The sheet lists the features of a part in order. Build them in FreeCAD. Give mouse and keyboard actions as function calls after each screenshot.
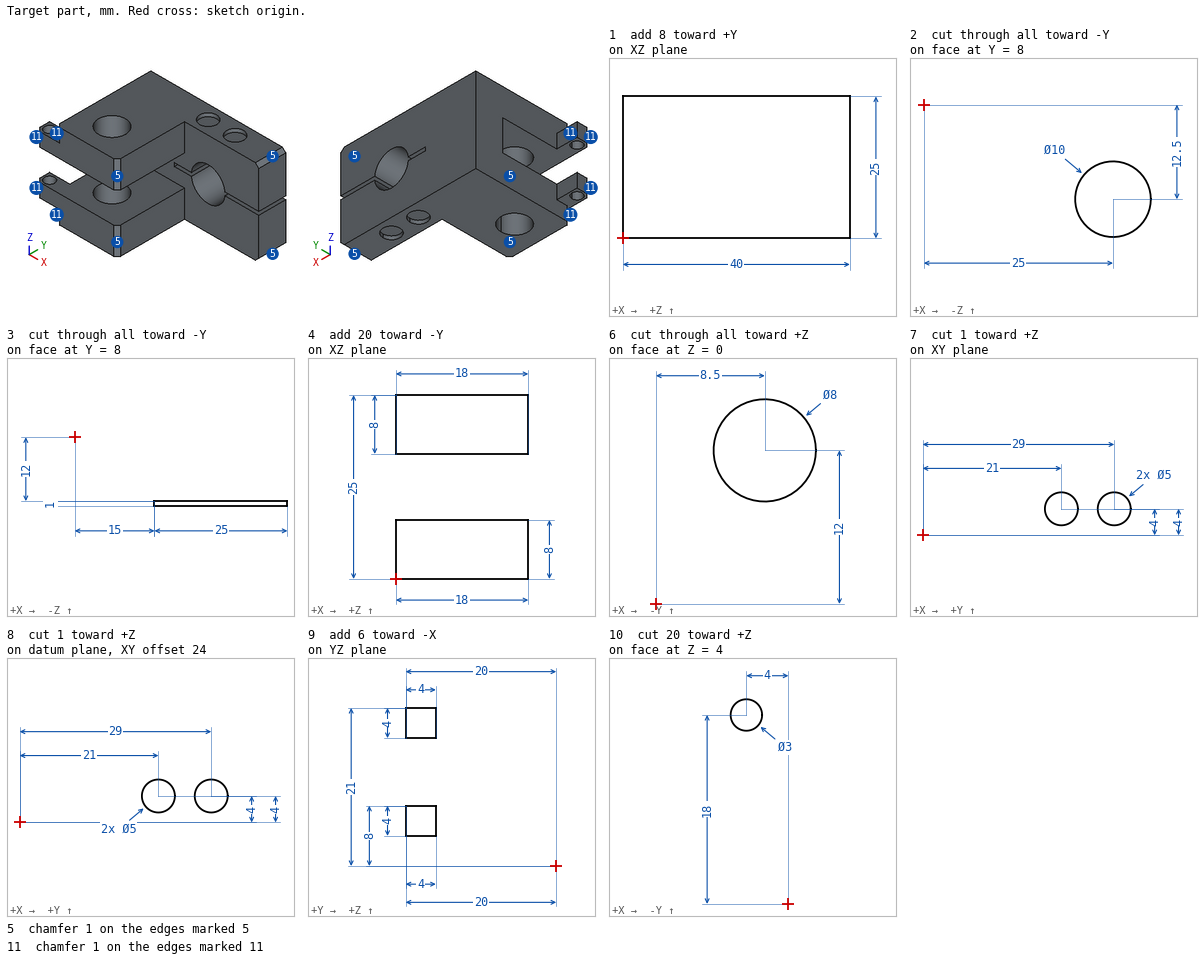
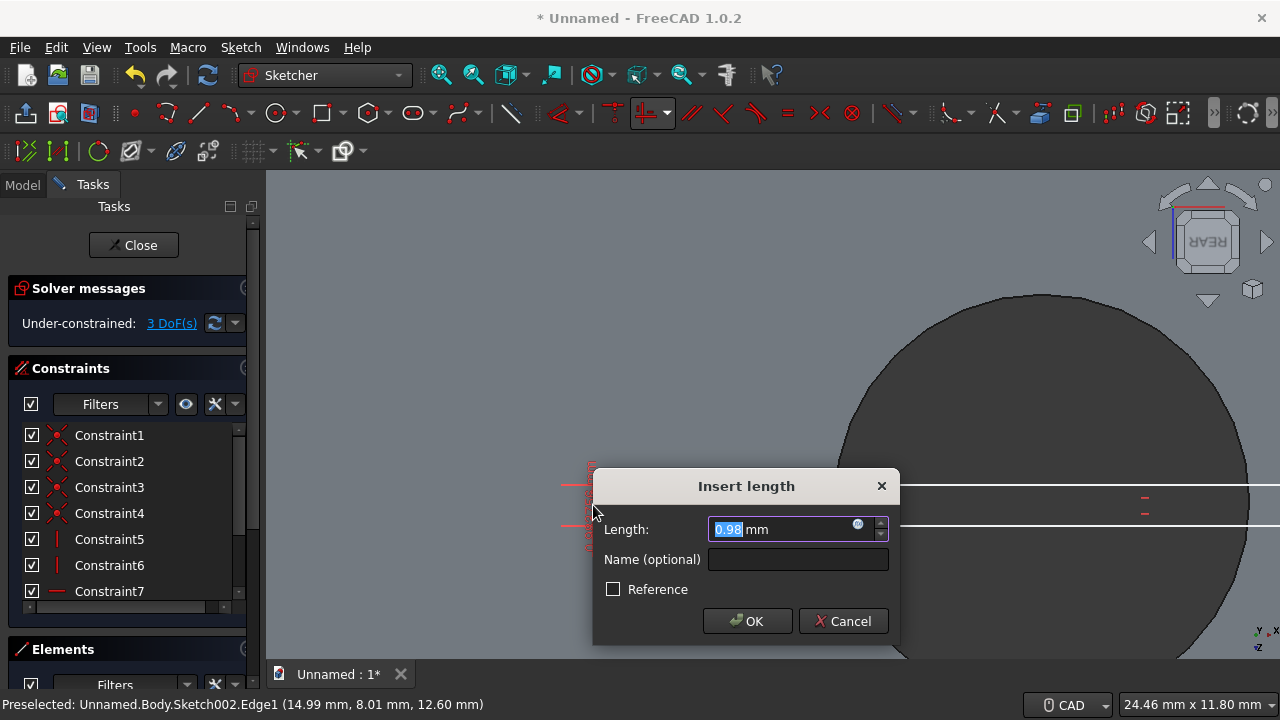
text(1)
key(Return)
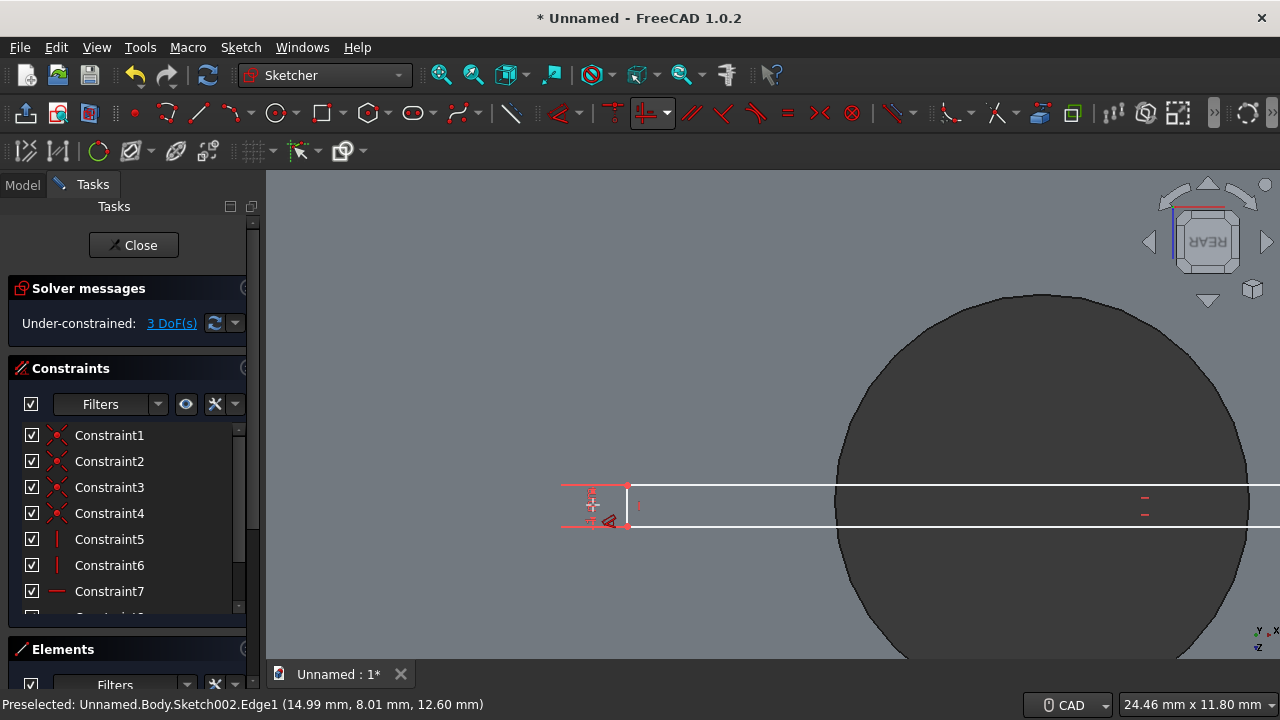
click(938, 527)
click(871, 561)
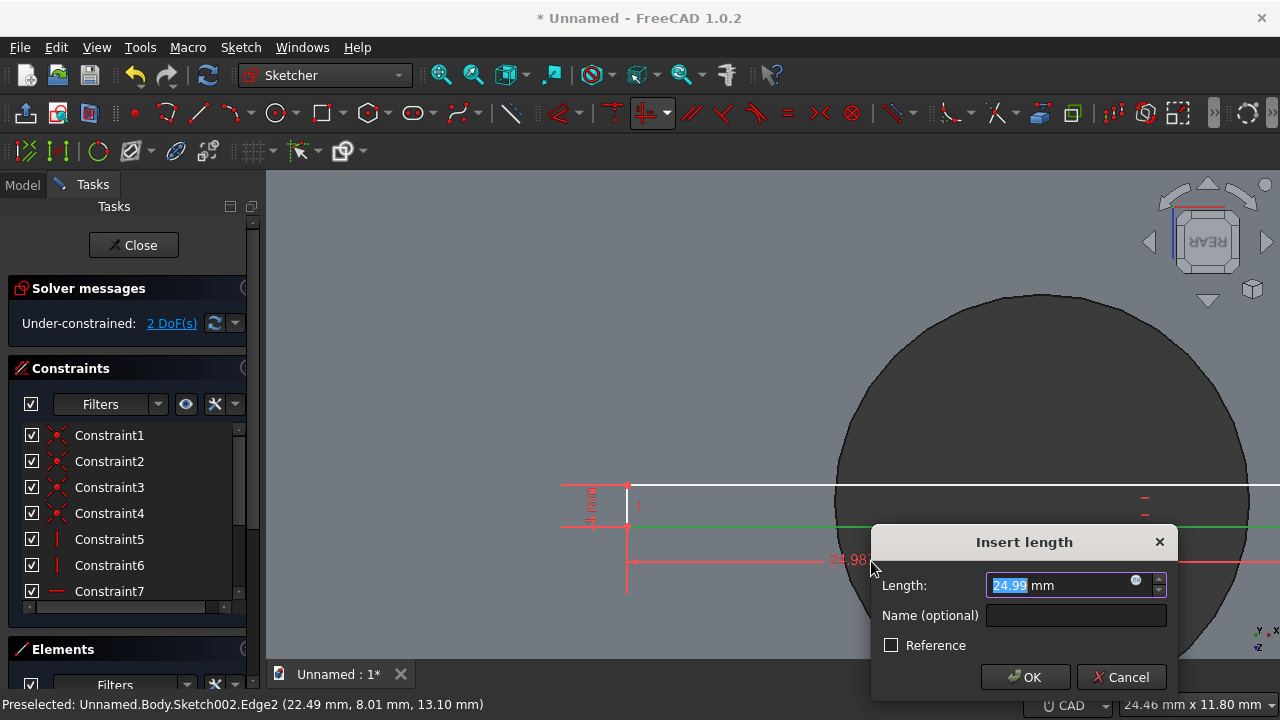
text(25)
key(Return)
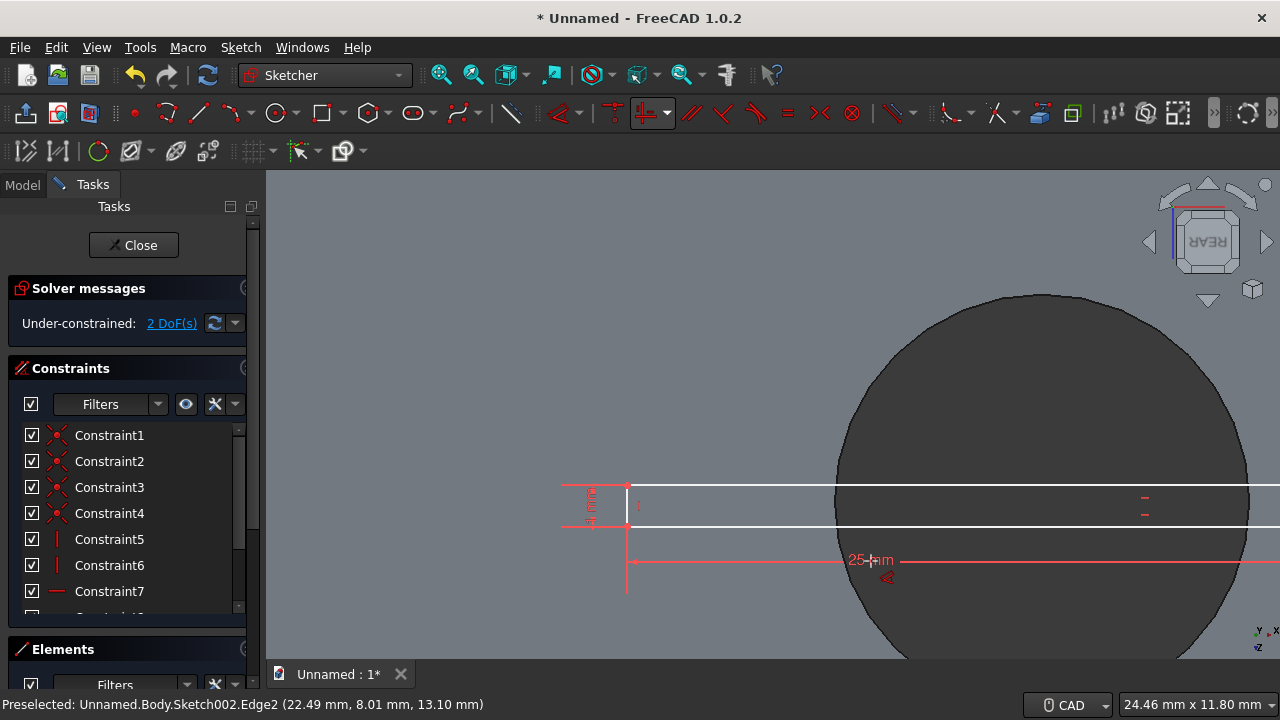
click(627, 485)
click(461, 519)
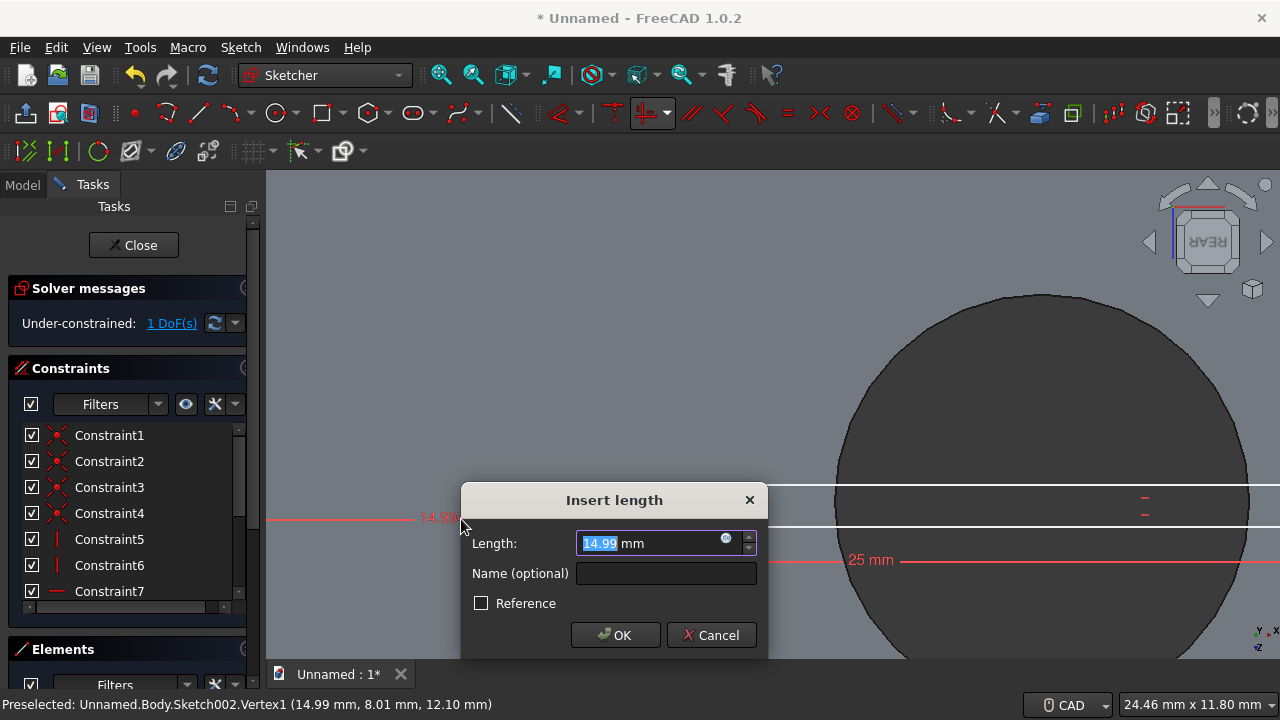
text(15)
key(Return)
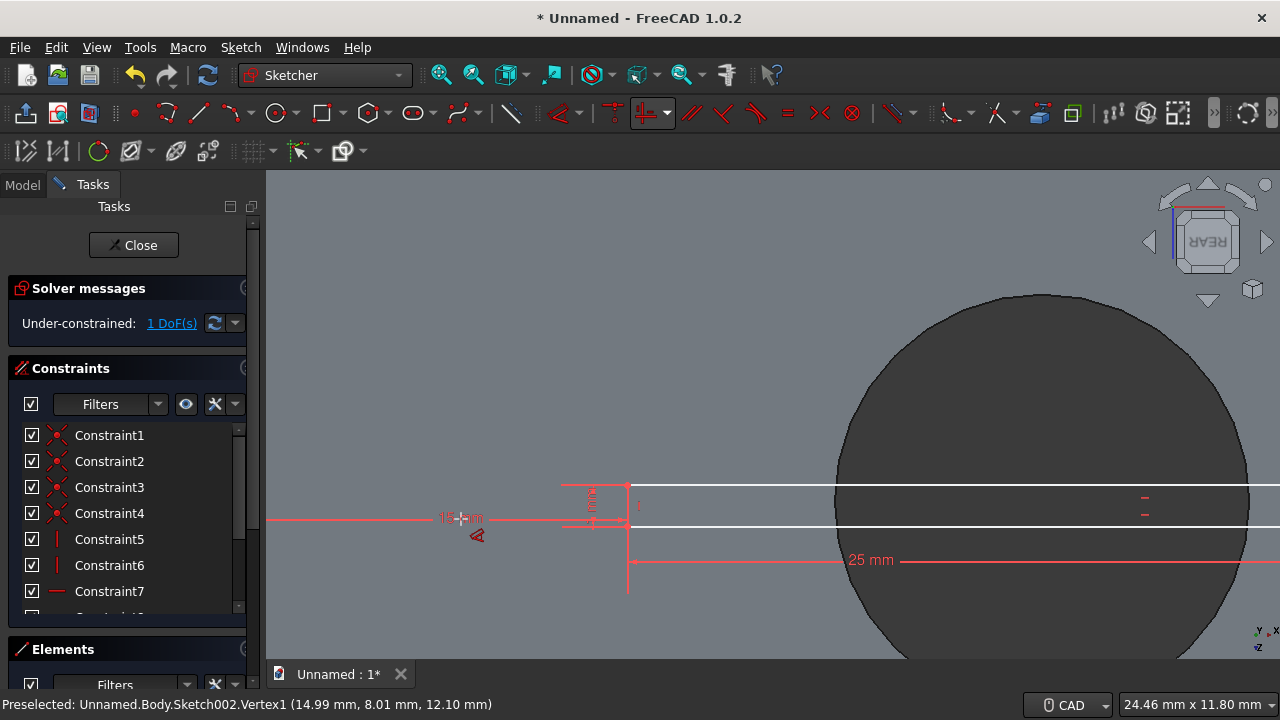
click(628, 485)
click(662, 342)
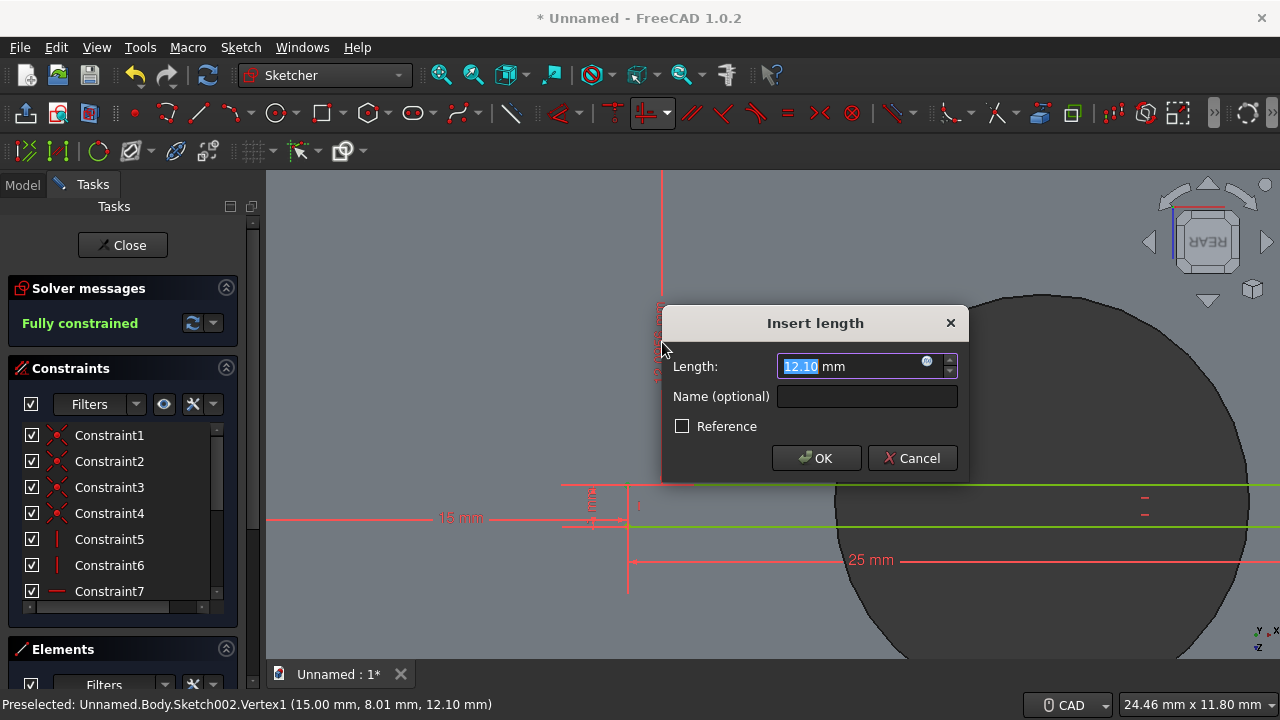
text(12)
key(Return)
key(Escape)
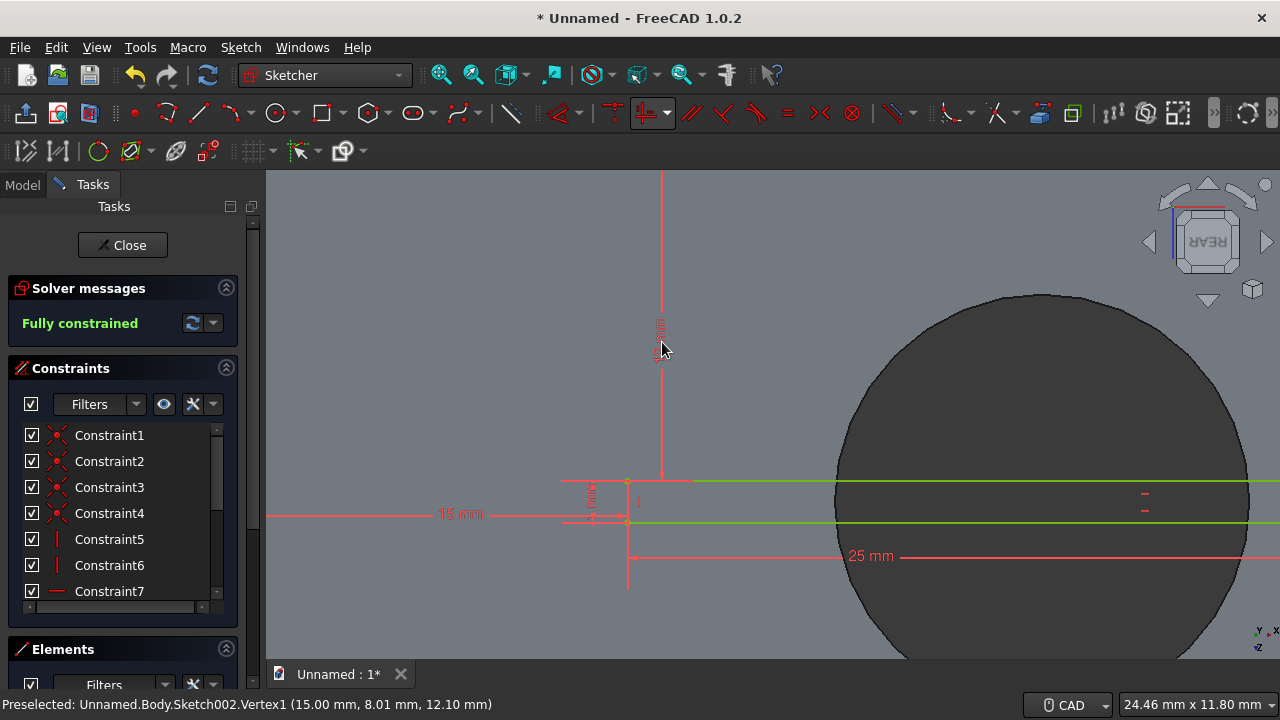
click(123, 245)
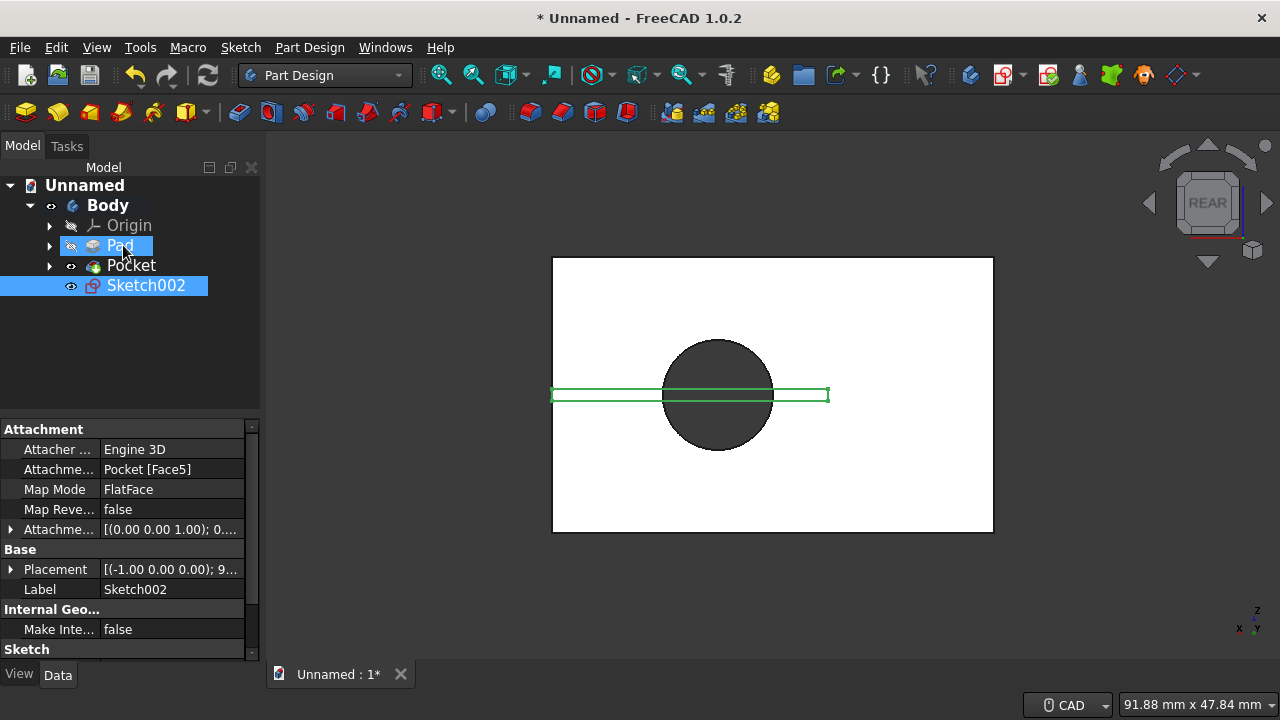
click(240, 112)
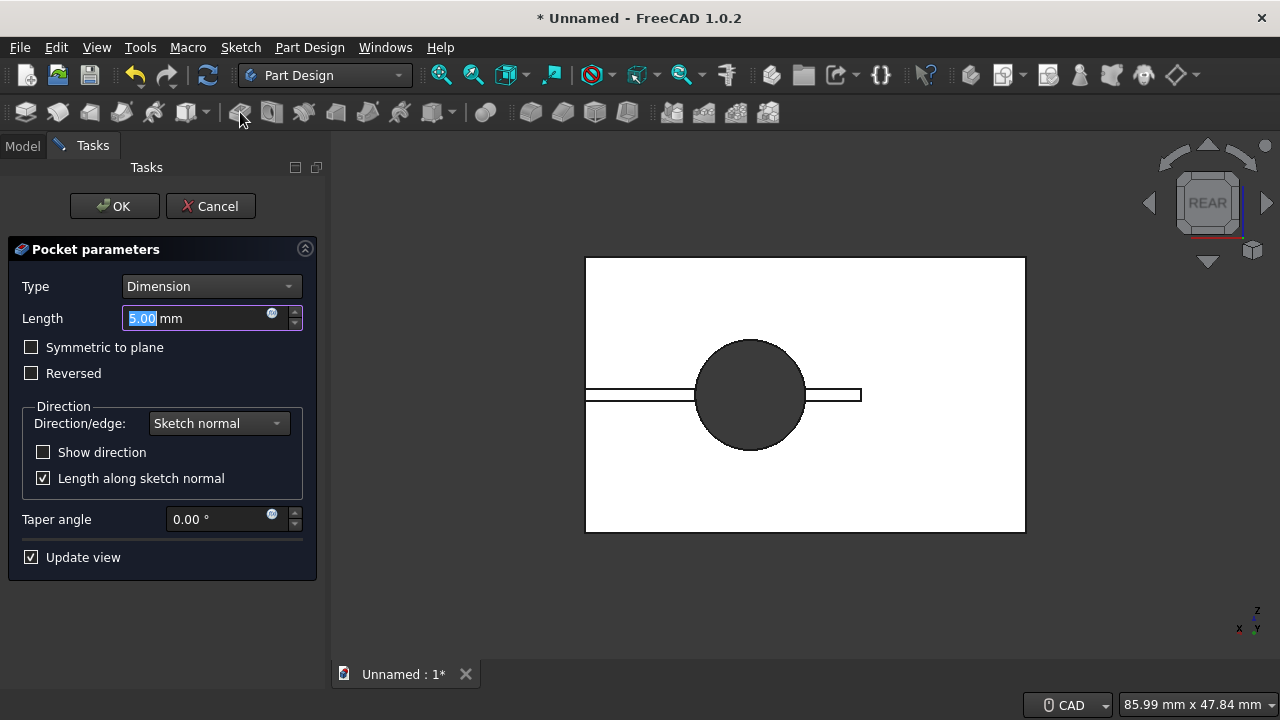
click(212, 286)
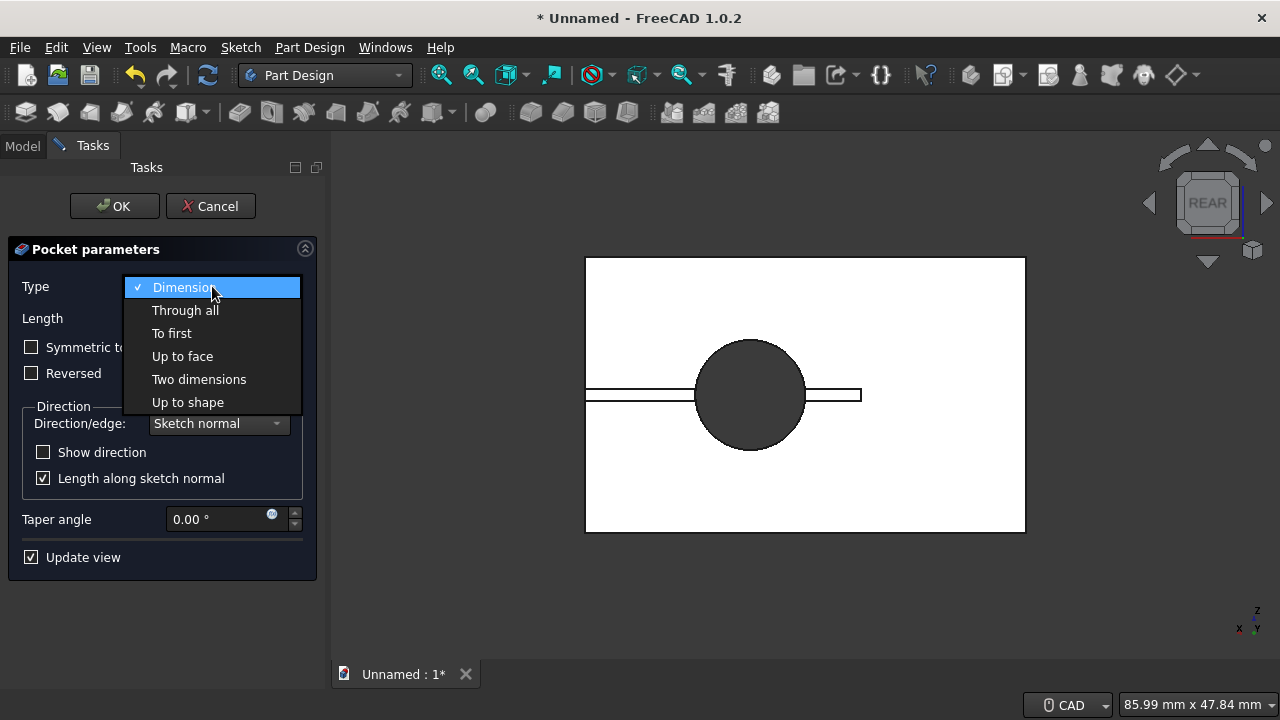
click(212, 310)